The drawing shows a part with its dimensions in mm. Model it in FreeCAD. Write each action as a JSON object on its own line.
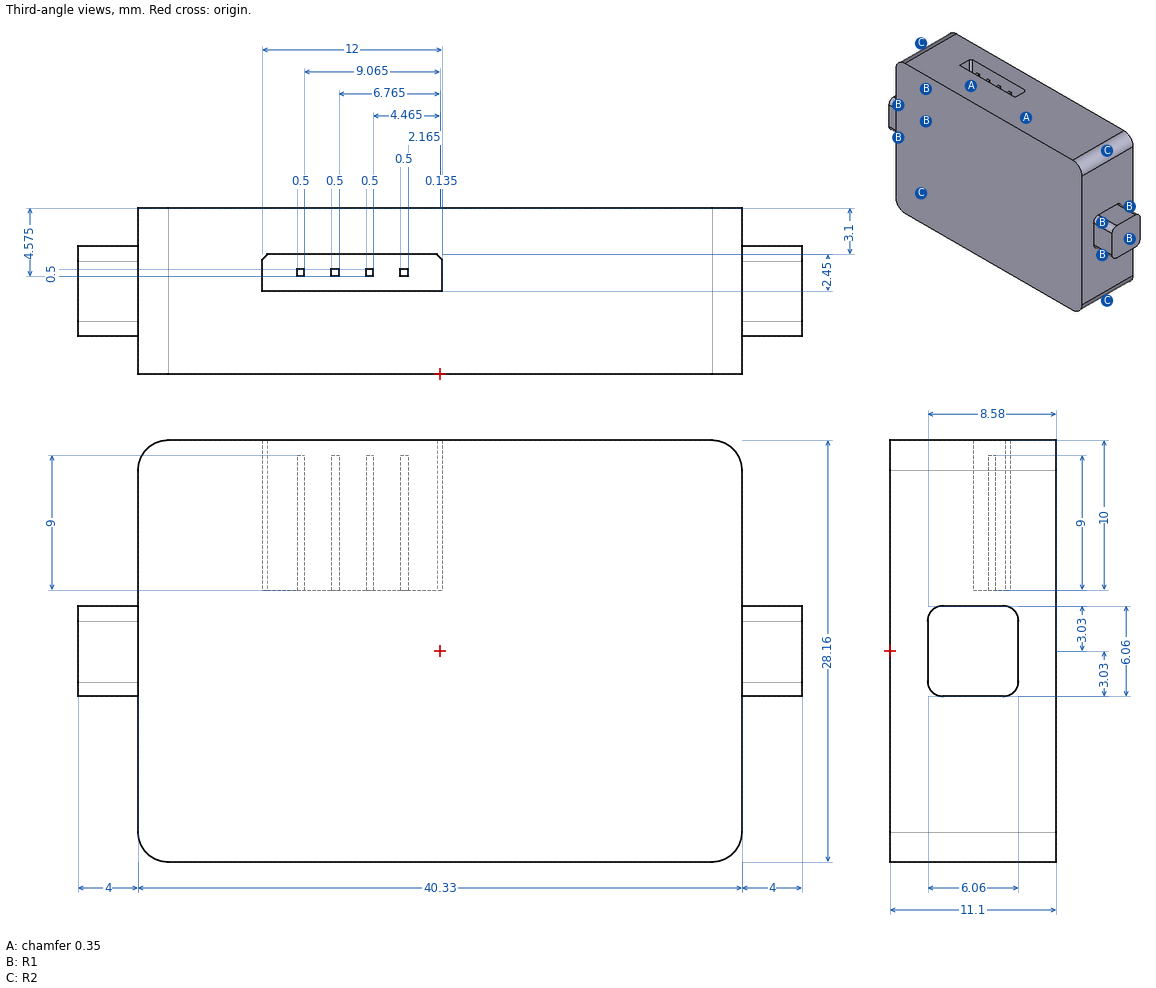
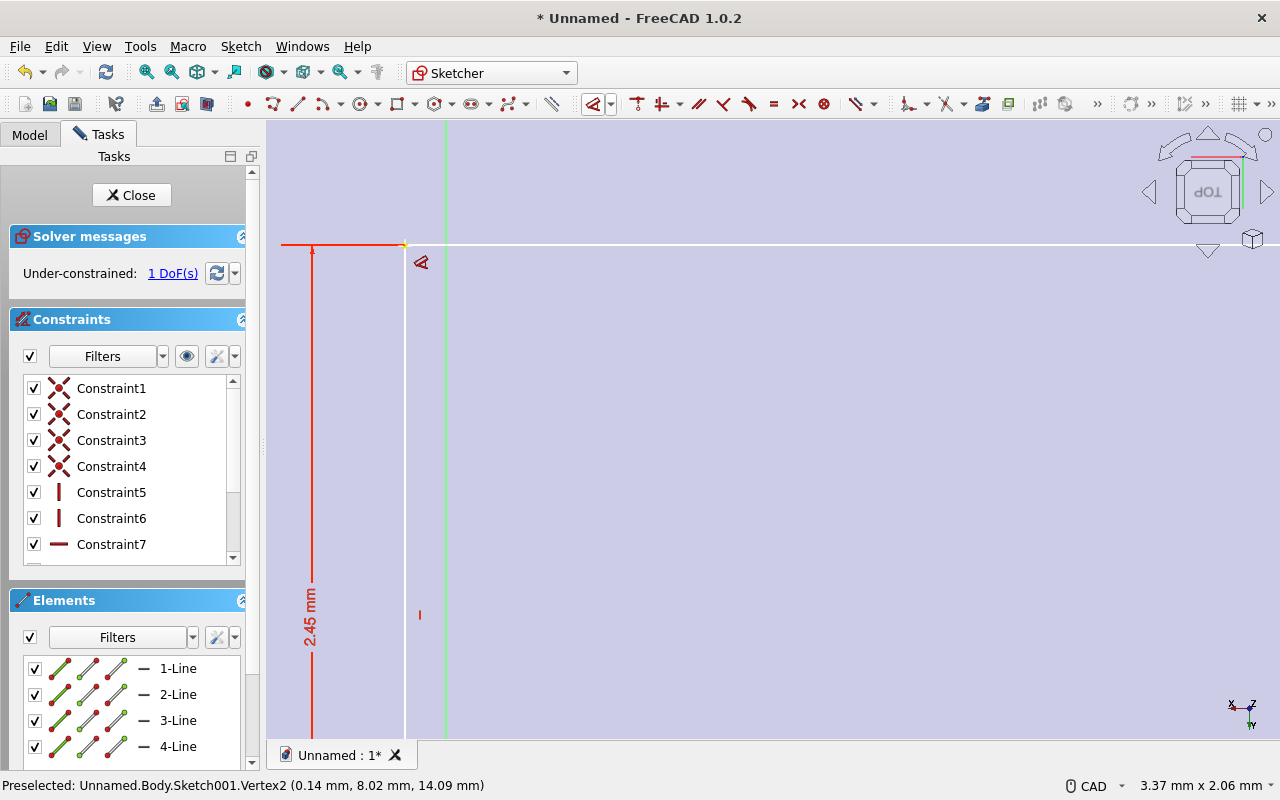
{"action": "left_click", "coordinate": [405, 245]}
{"action": "left_click", "coordinate": [426, 211]}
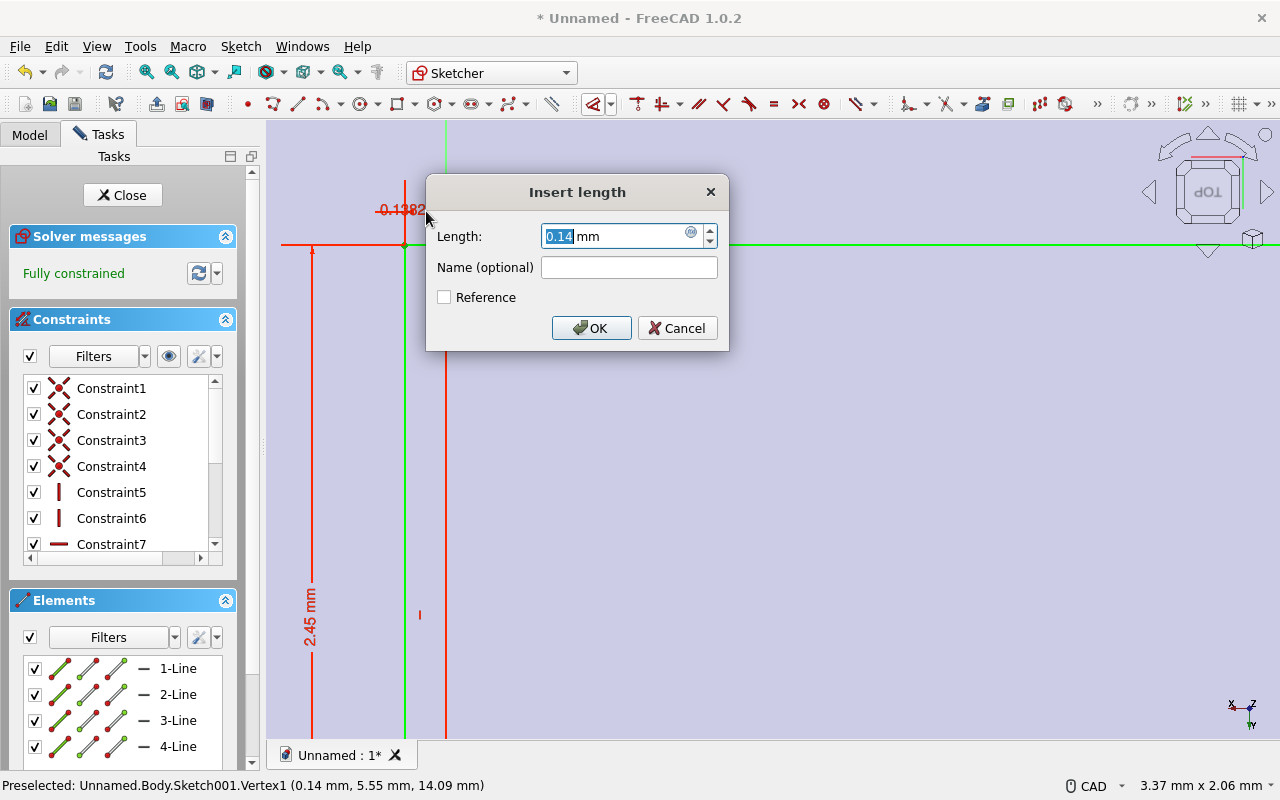
{"action": "type", "text": "0.135"}
{"action": "key", "text": "Return"}
{"action": "key", "text": "Escape"}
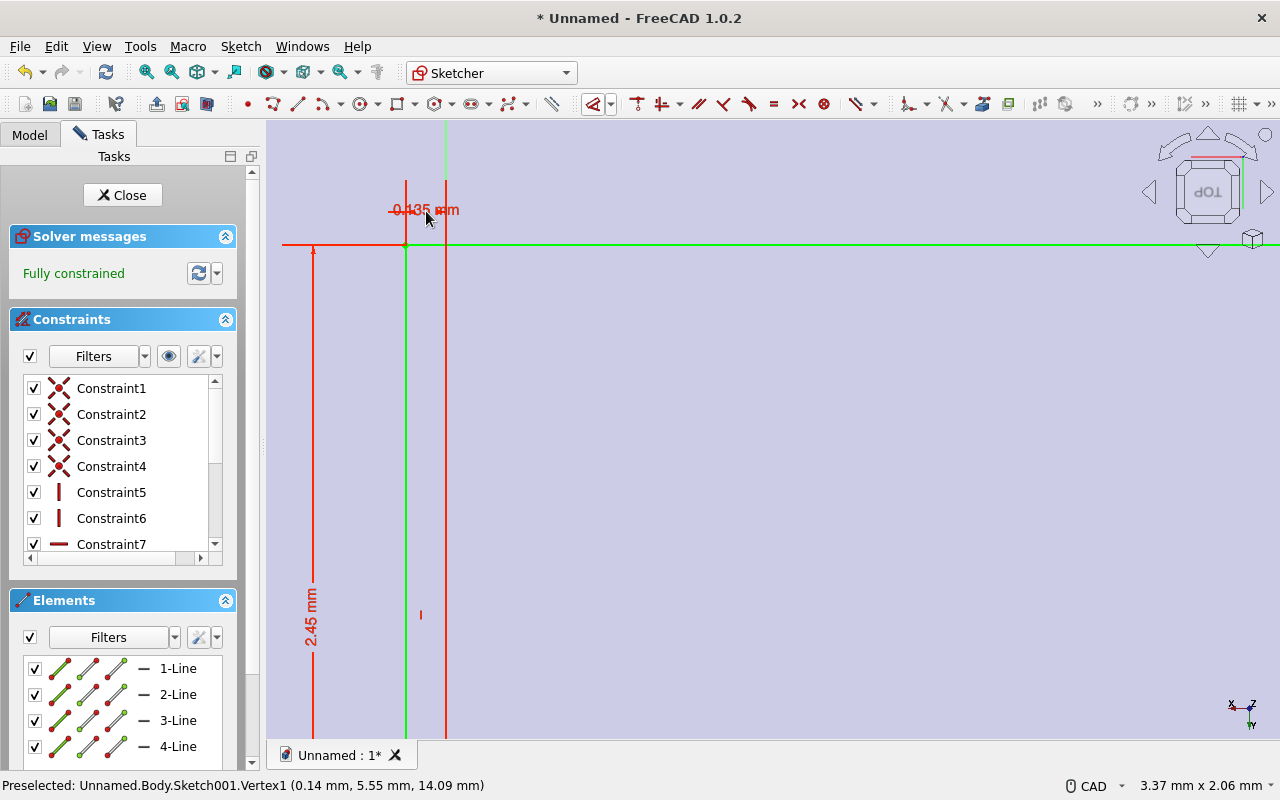
{"action": "left_click", "coordinate": [123, 195]}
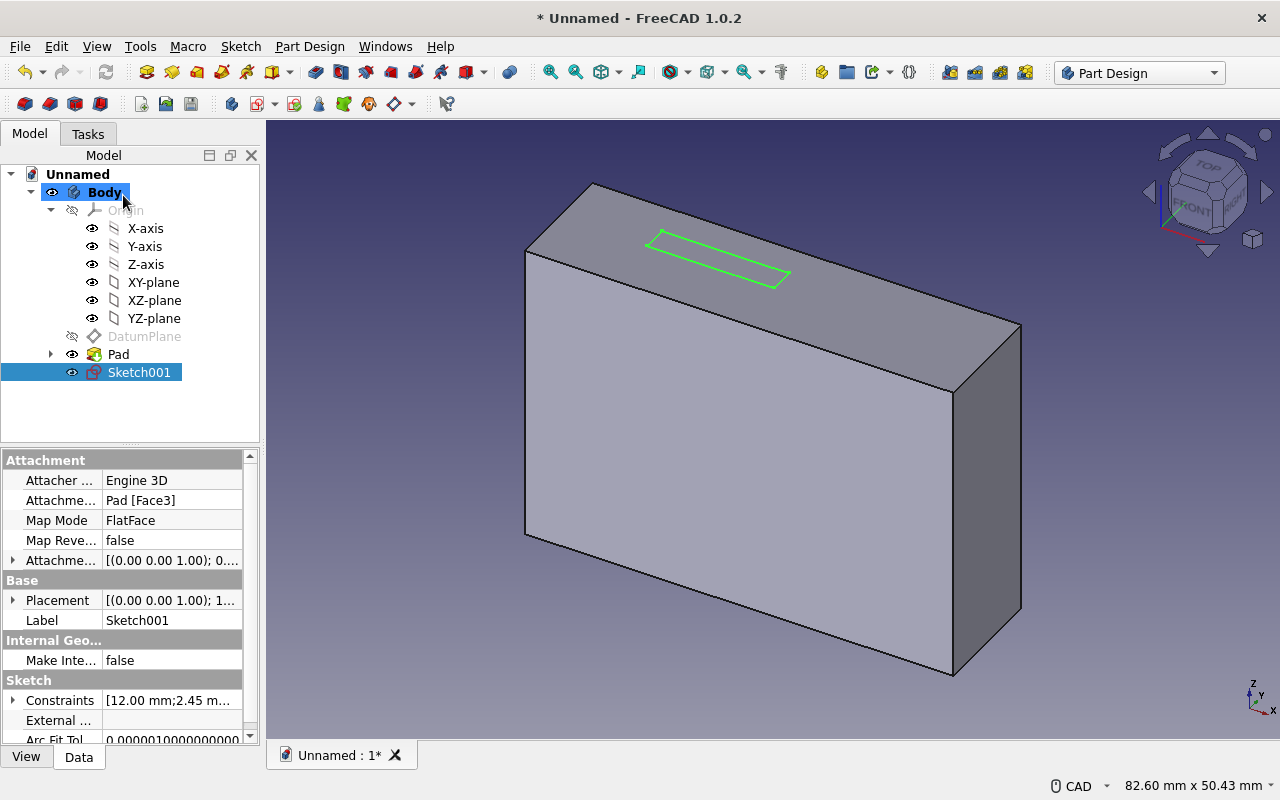
{"action": "left_click", "coordinate": [316, 72]}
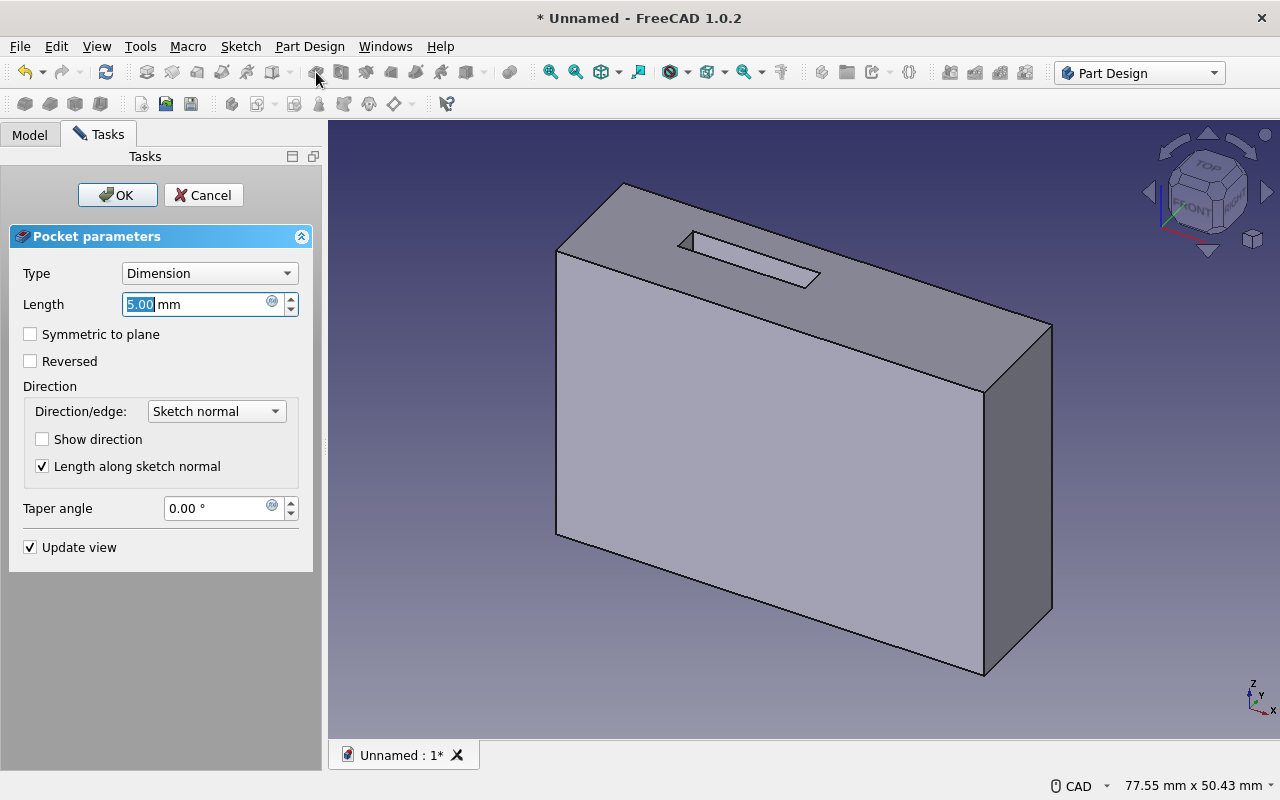
{"action": "type", "text": "10"}
{"action": "key", "text": "Tab"}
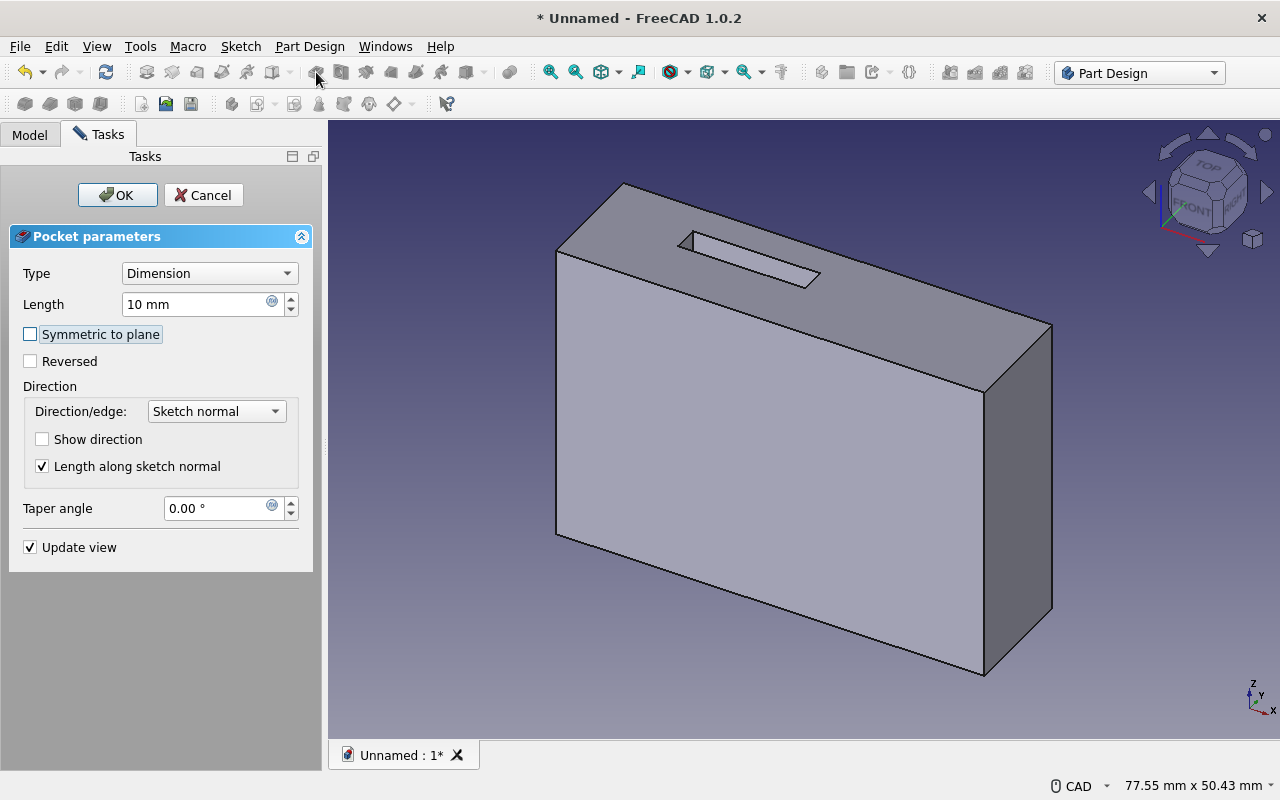
{"action": "left_click", "coordinate": [118, 195]}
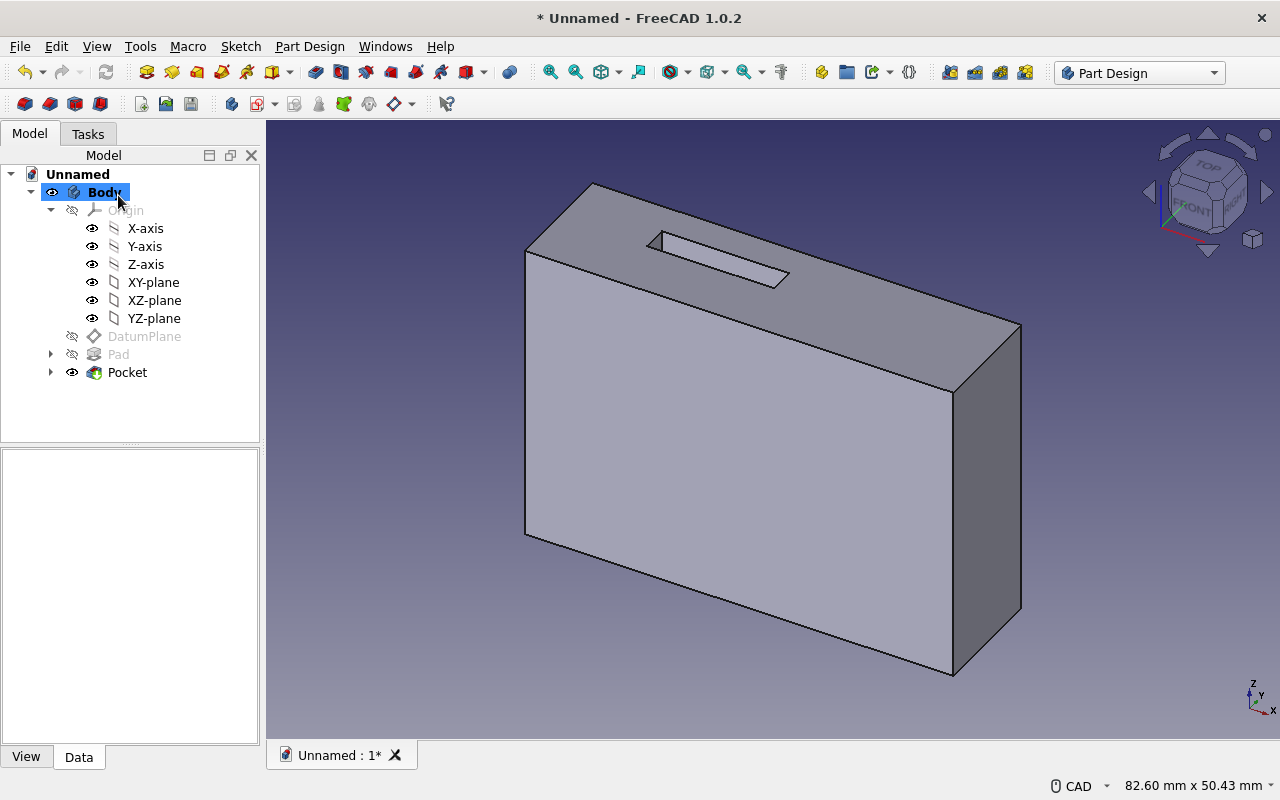
{"action": "key", "text": "0"}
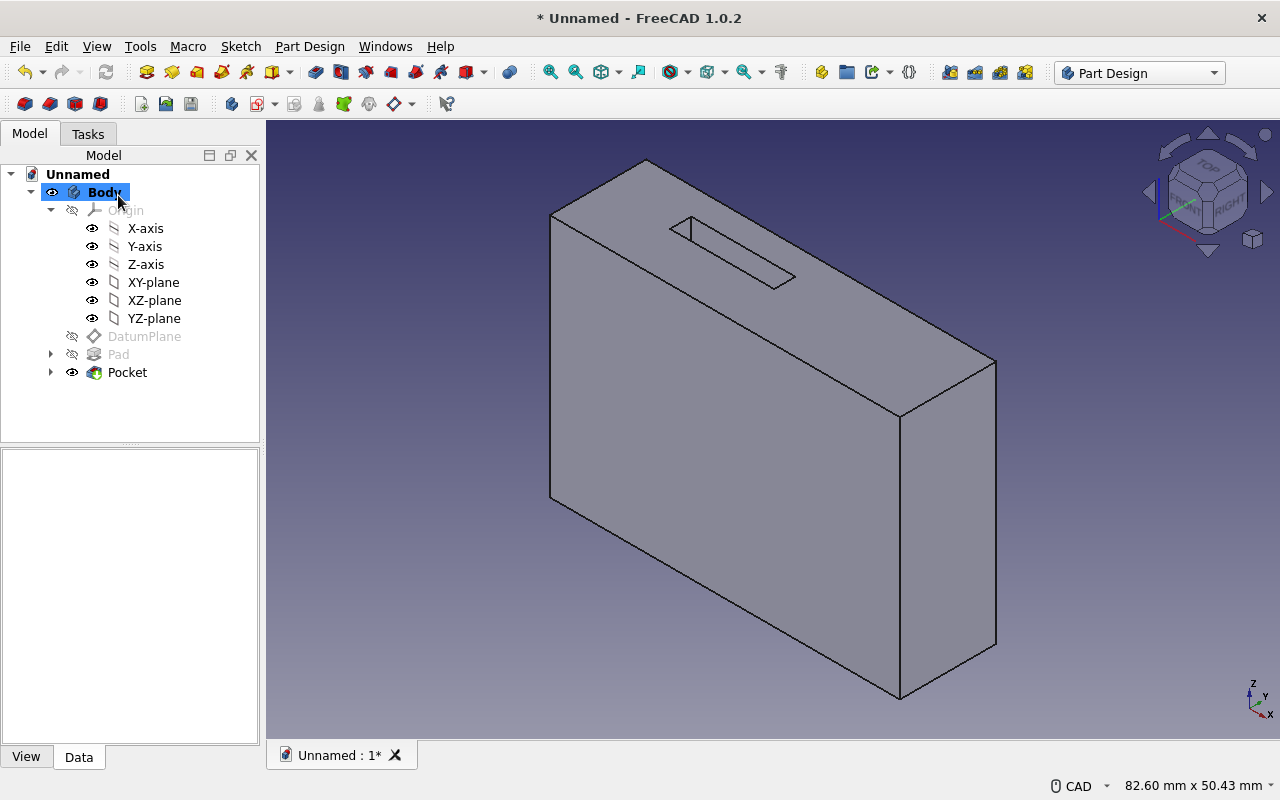
{"action": "key", "text": "2"}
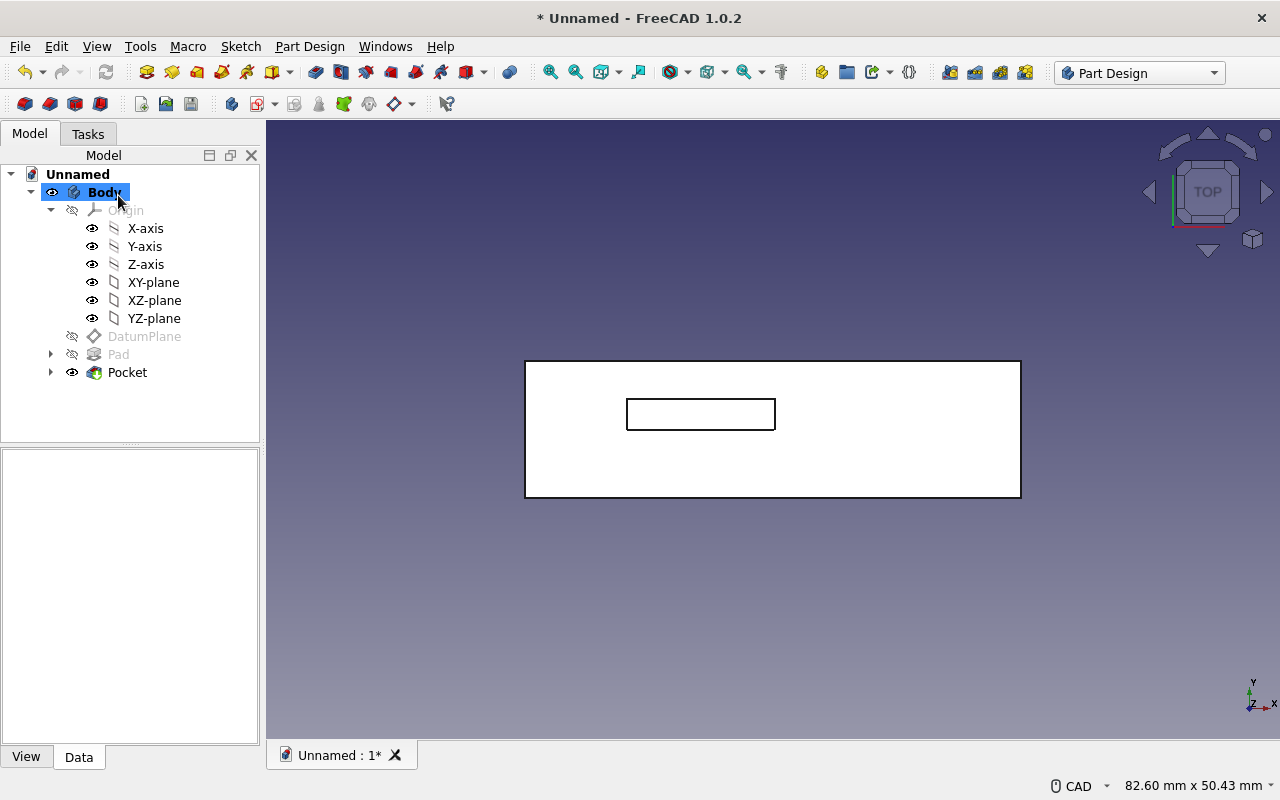
{"action": "left_click", "coordinate": [743, 413]}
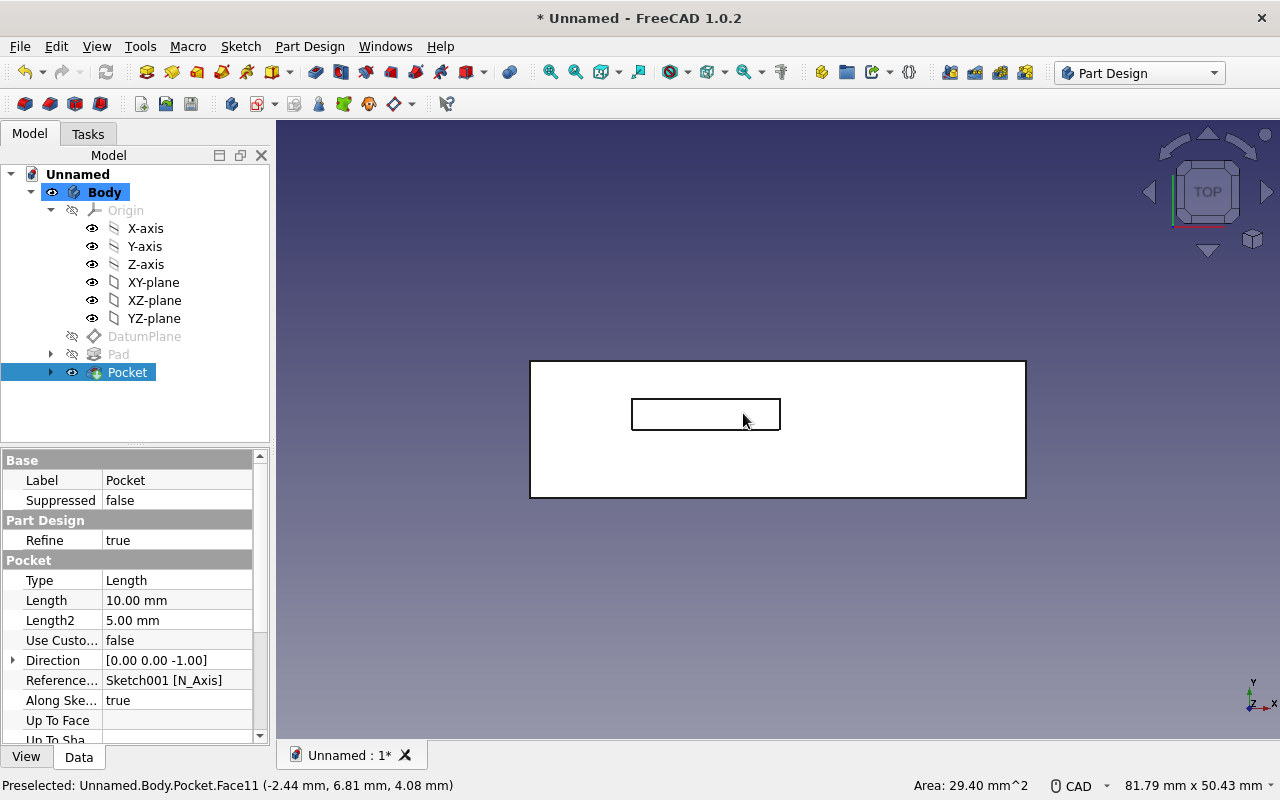
{"action": "left_click", "coordinate": [256, 104]}